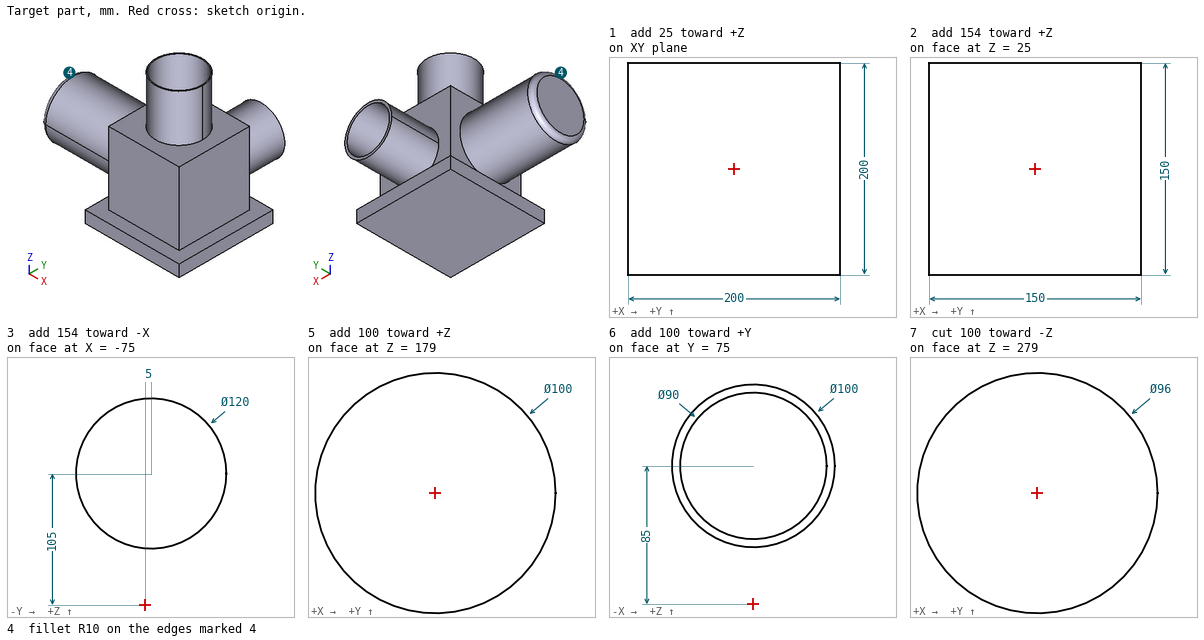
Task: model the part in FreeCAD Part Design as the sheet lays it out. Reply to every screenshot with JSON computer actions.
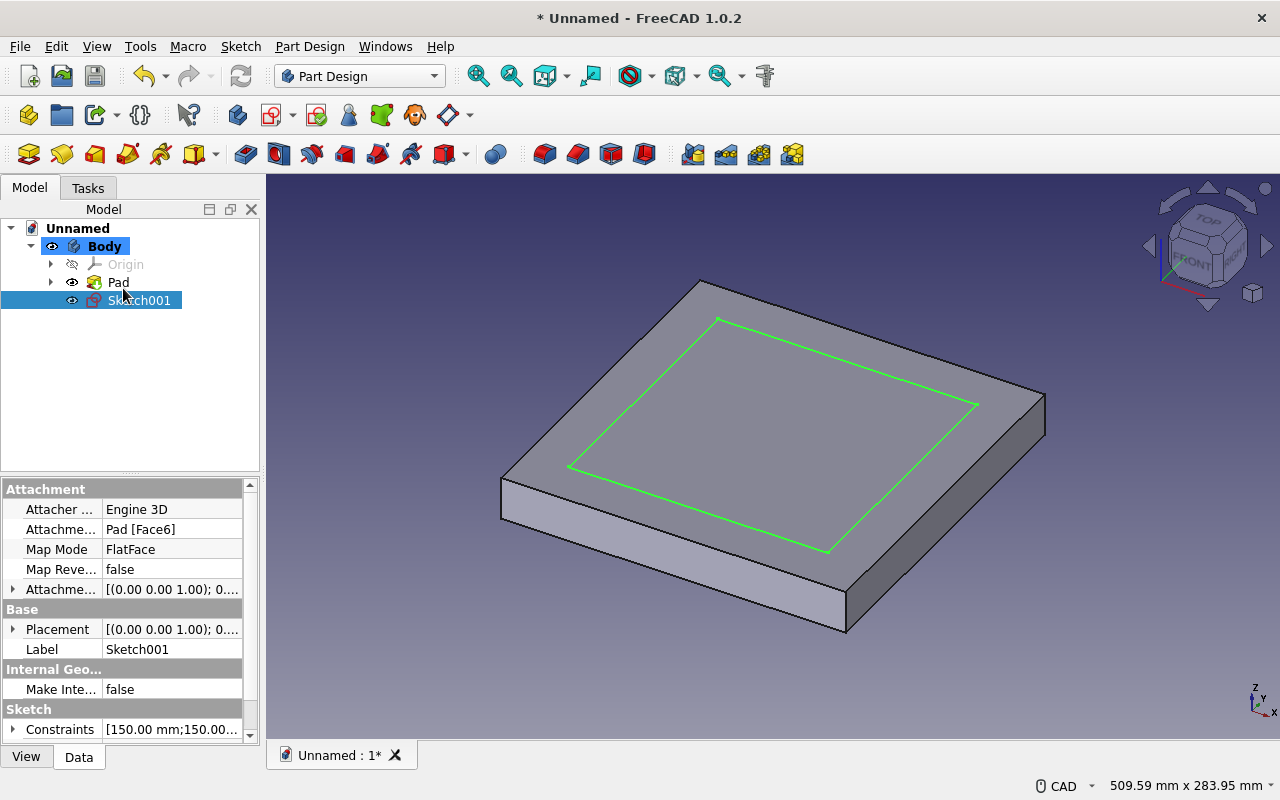
{"action": "left_click", "coordinate": [29, 154]}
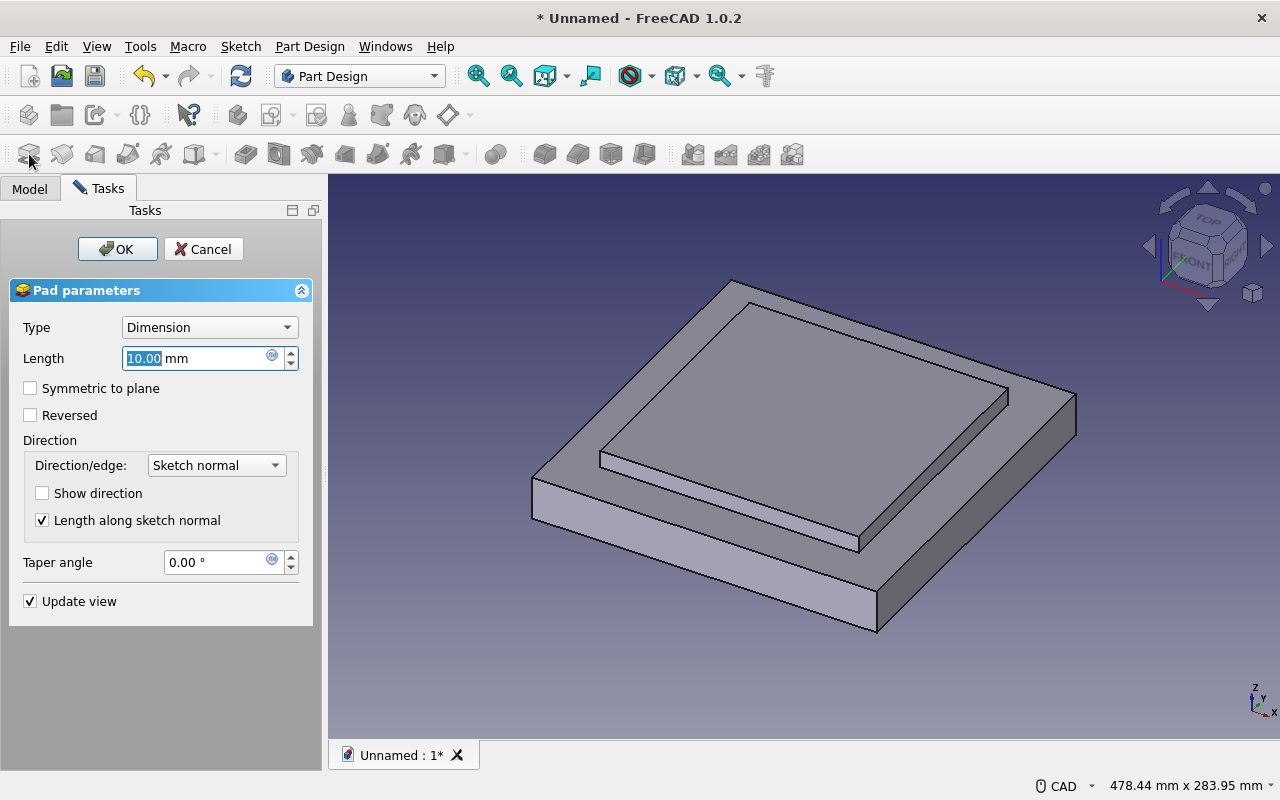
{"action": "type", "text": "154"}
{"action": "key", "text": "Tab"}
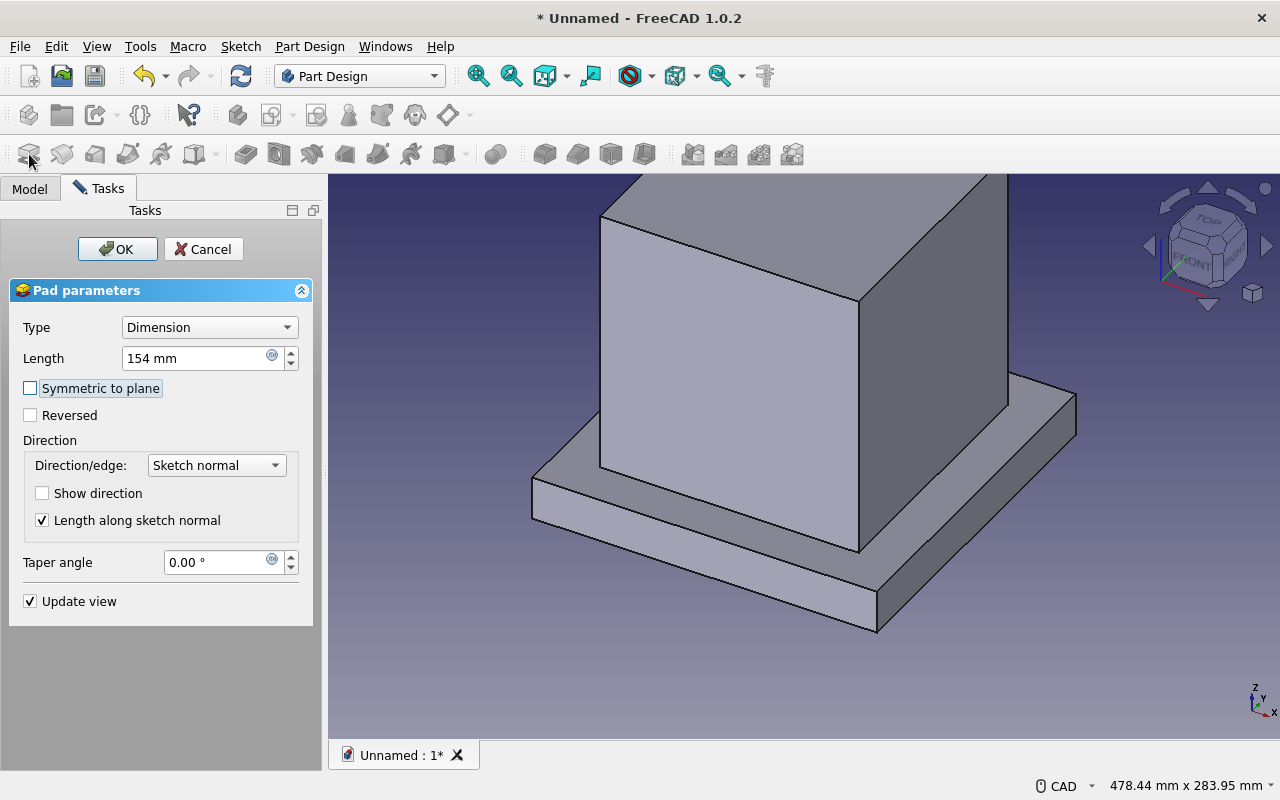
{"action": "left_click", "coordinate": [118, 249]}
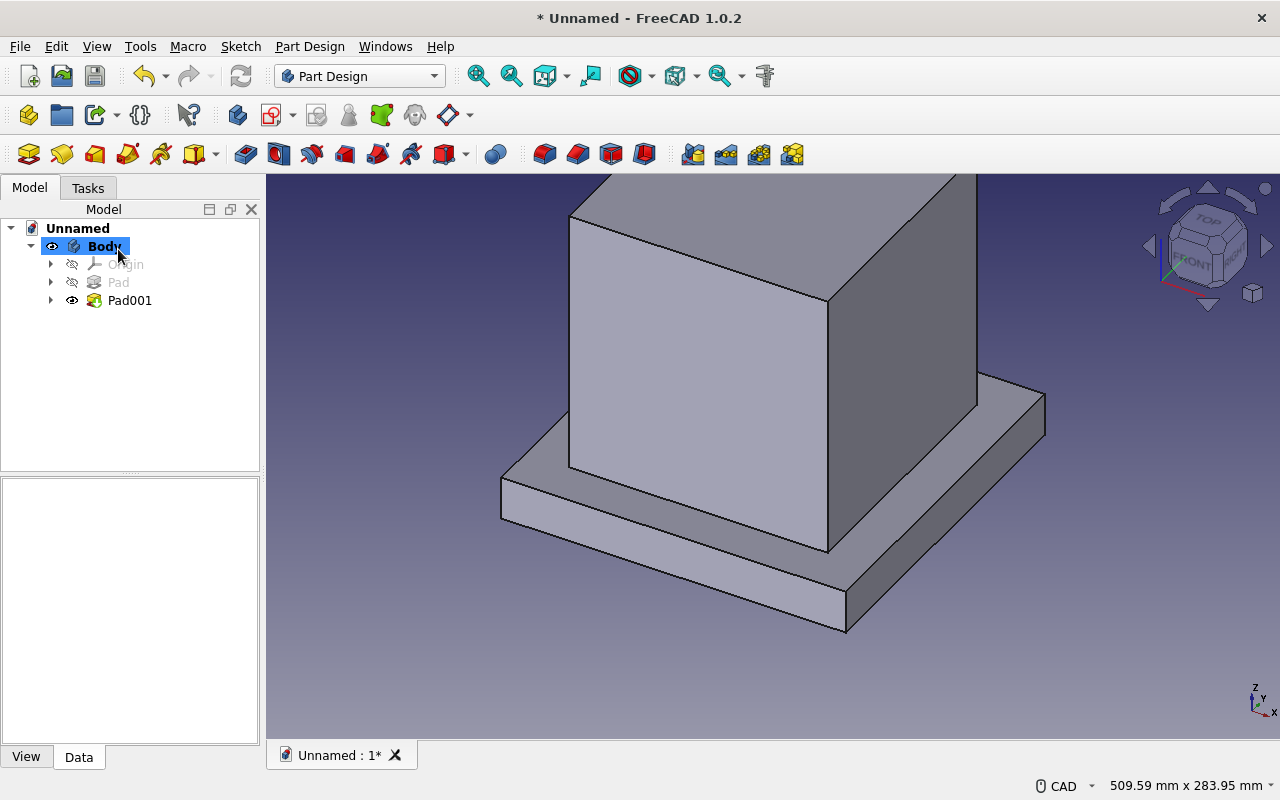
{"action": "left_click", "coordinate": [479, 76]}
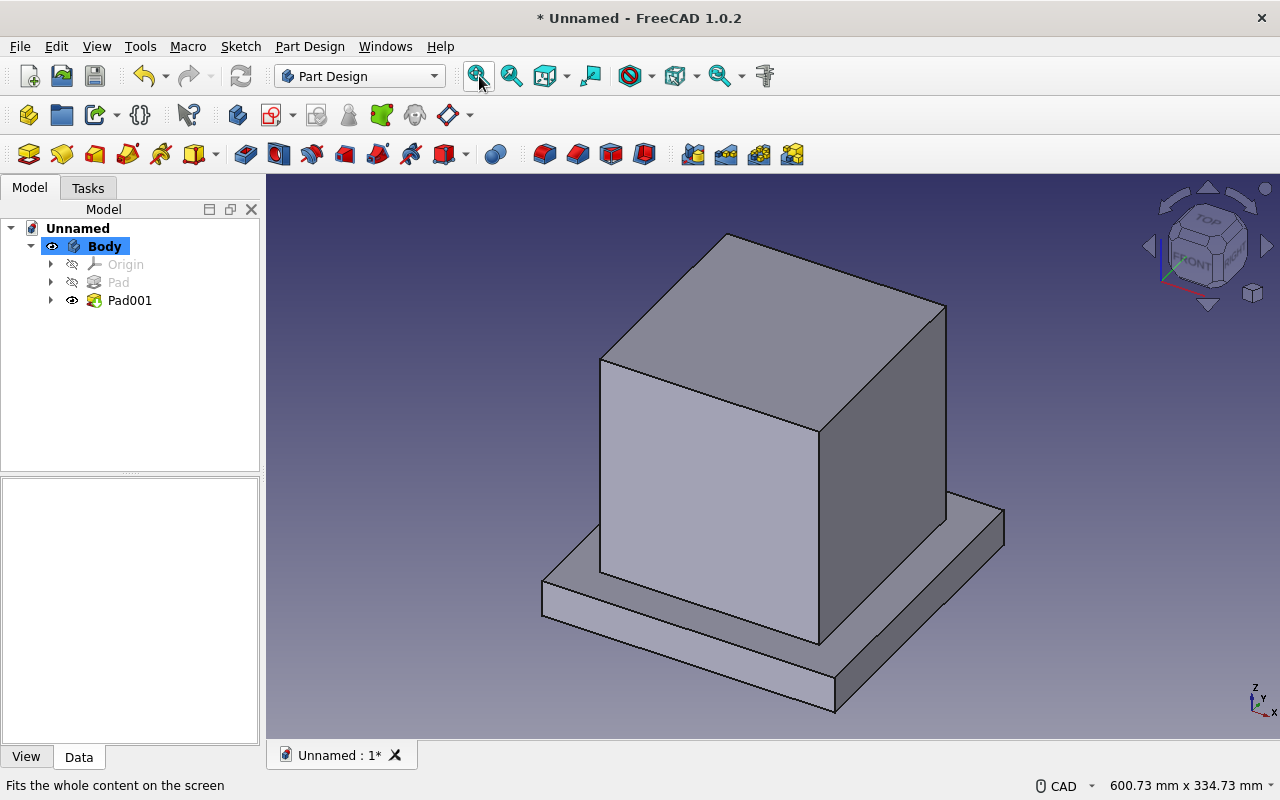
{"action": "key", "text": "6"}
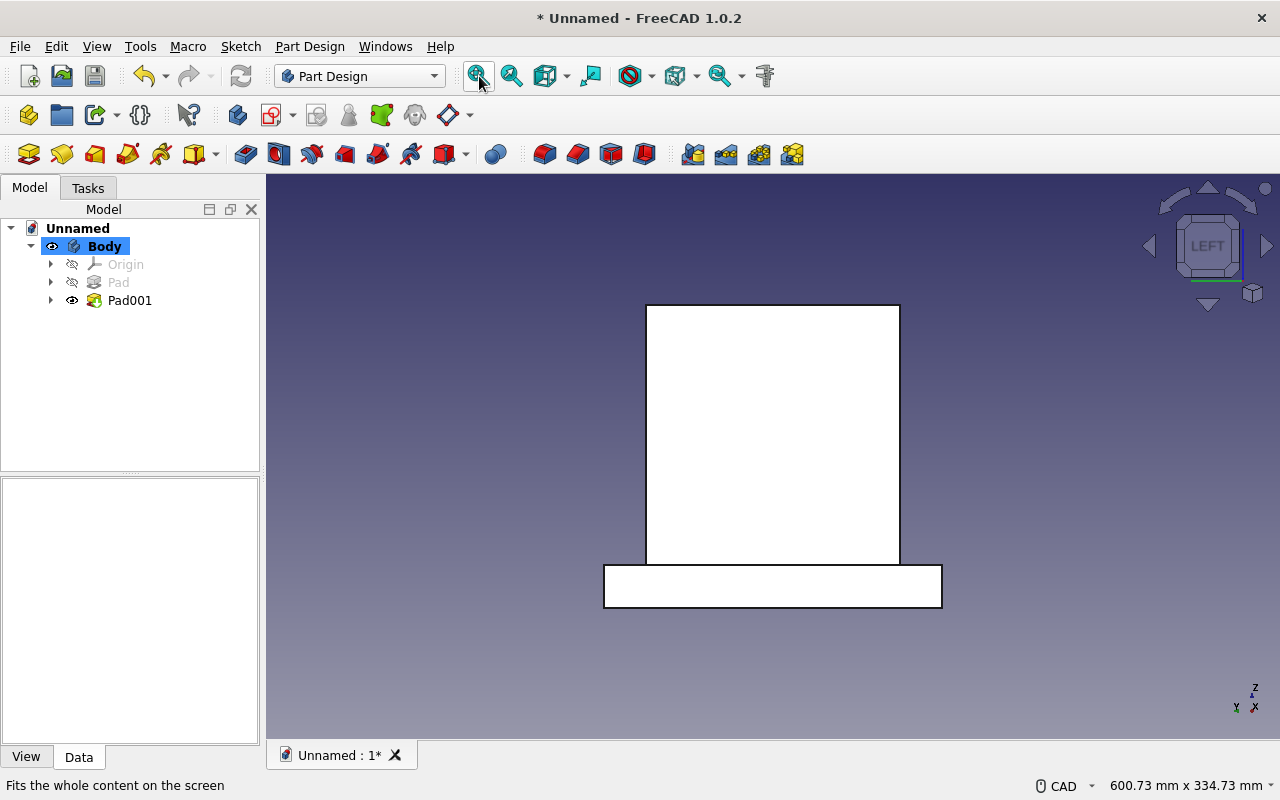
{"action": "left_click", "coordinate": [773, 434]}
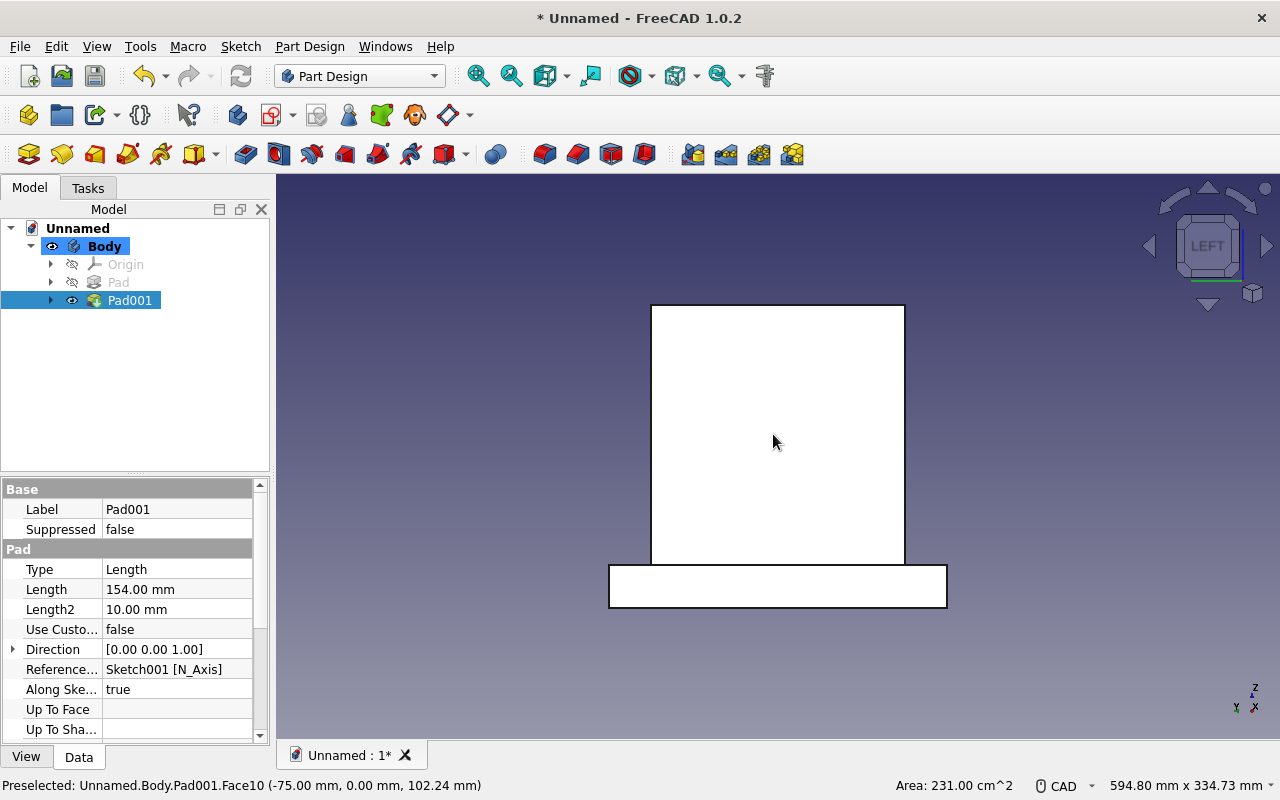
{"action": "left_click", "coordinate": [270, 116]}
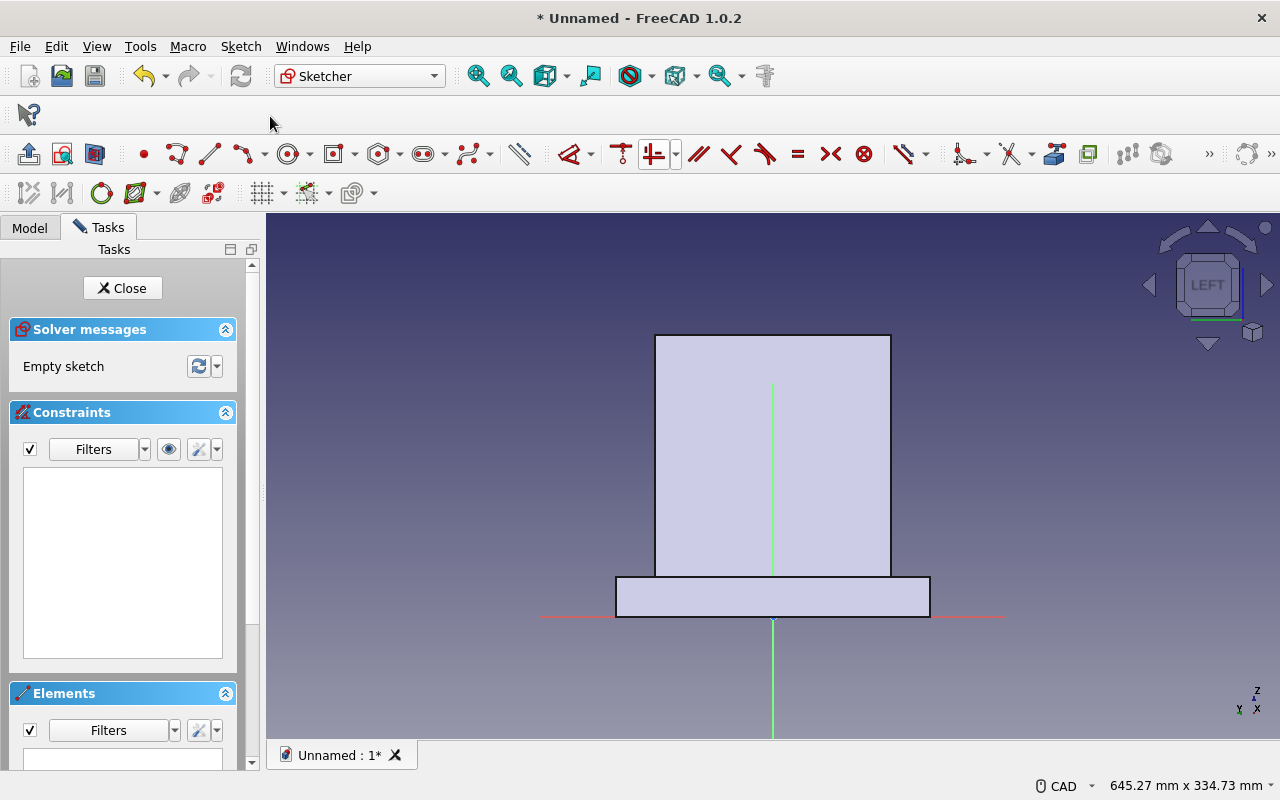
{"action": "left_click", "coordinate": [288, 154]}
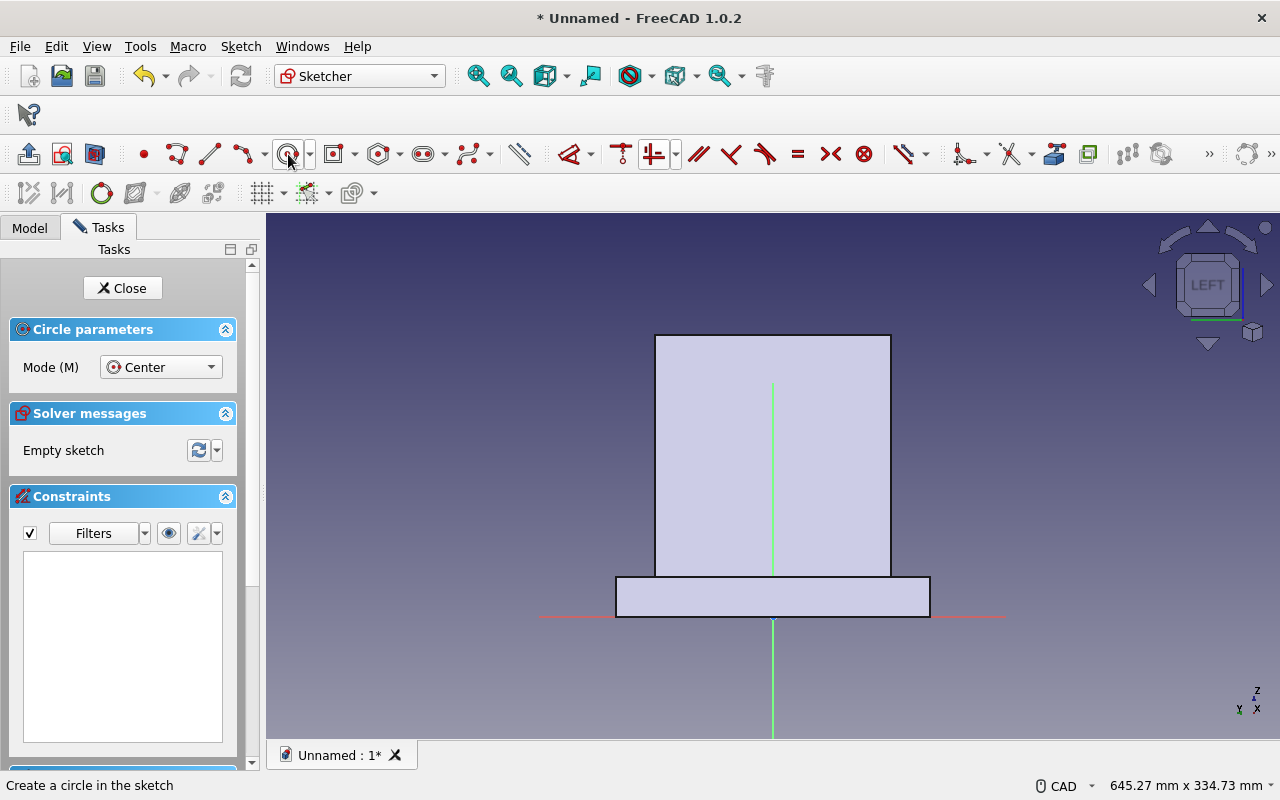
{"action": "scroll", "coordinate": [781, 452], "scroll_direction": "up", "scroll_amount": 4}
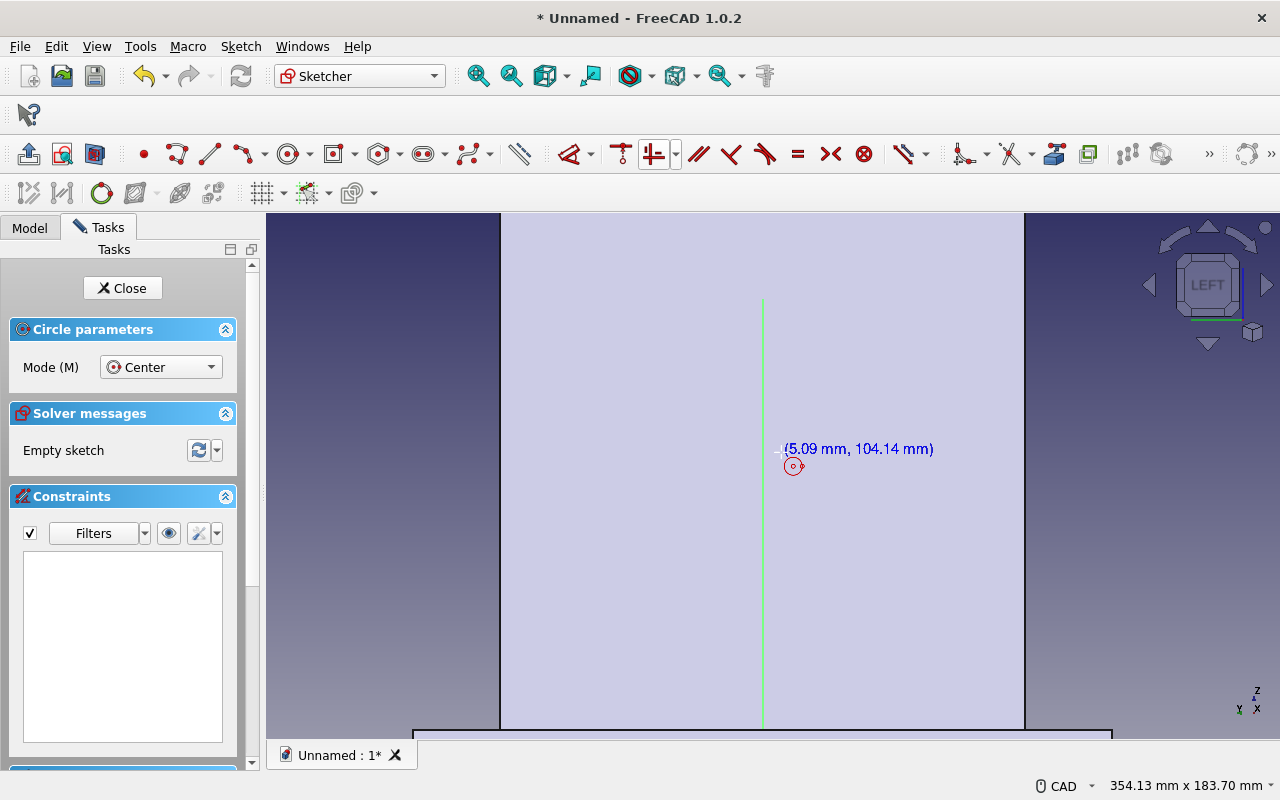
{"action": "left_click", "coordinate": [780, 451]}
{"action": "mouse_move", "coordinate": [928, 302]}